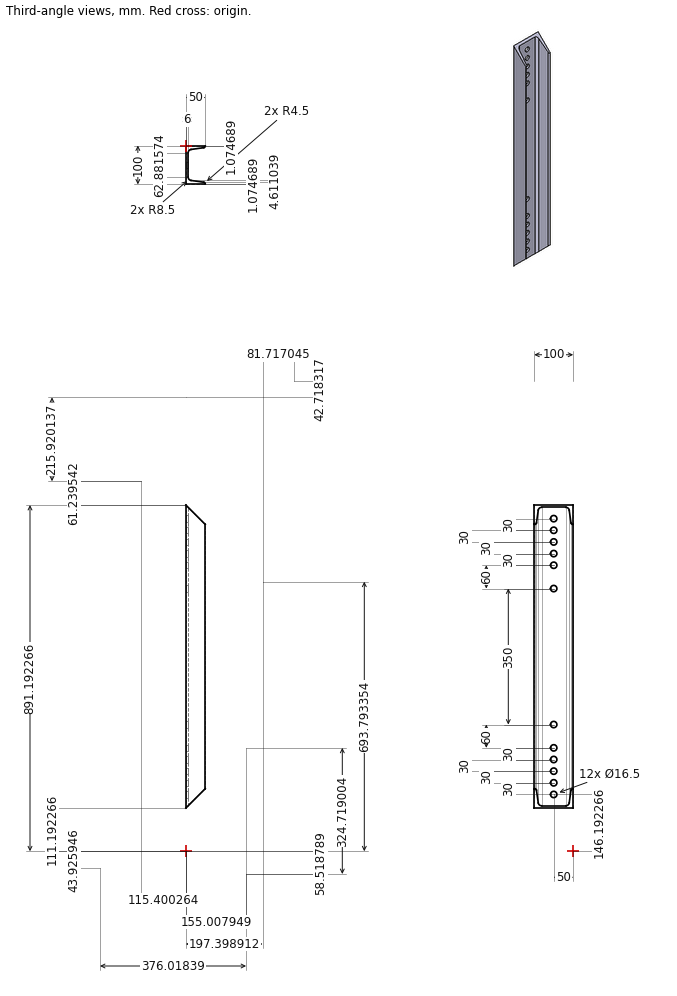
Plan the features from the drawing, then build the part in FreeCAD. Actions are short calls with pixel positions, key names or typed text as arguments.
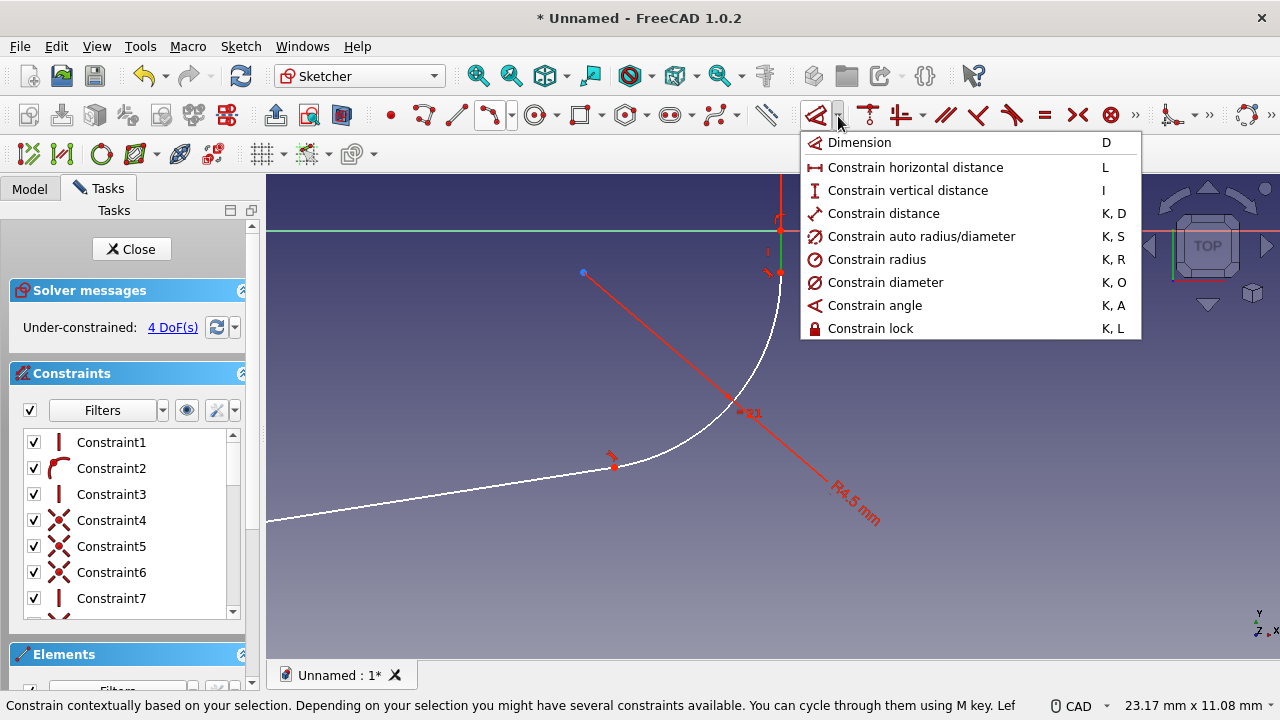
click(971, 190)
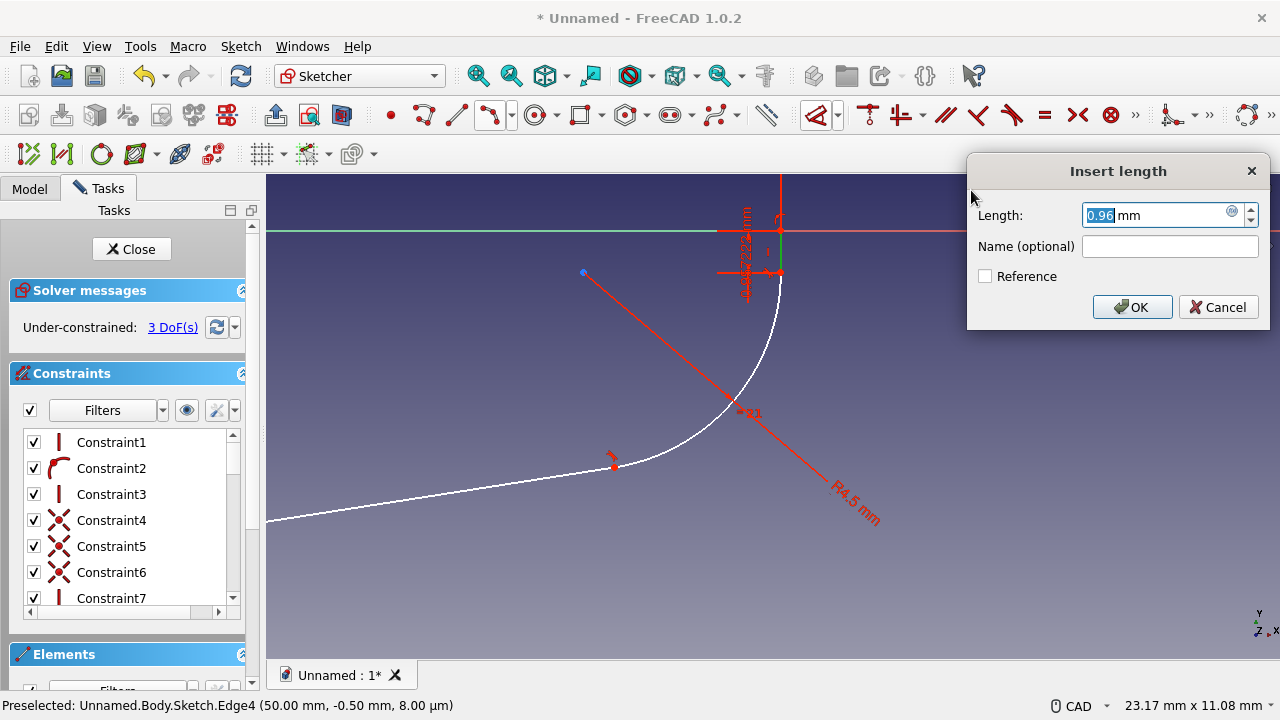
text(1.074689)
key(Return)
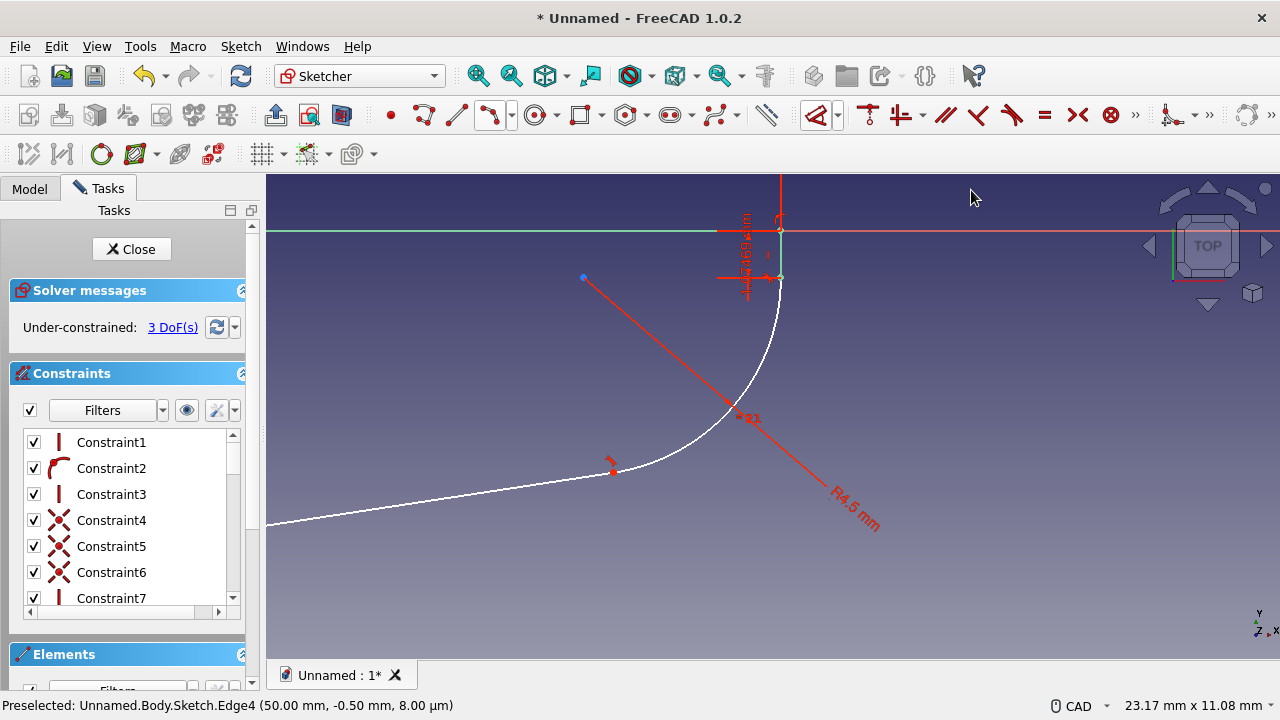
scroll(786, 256, down, 13)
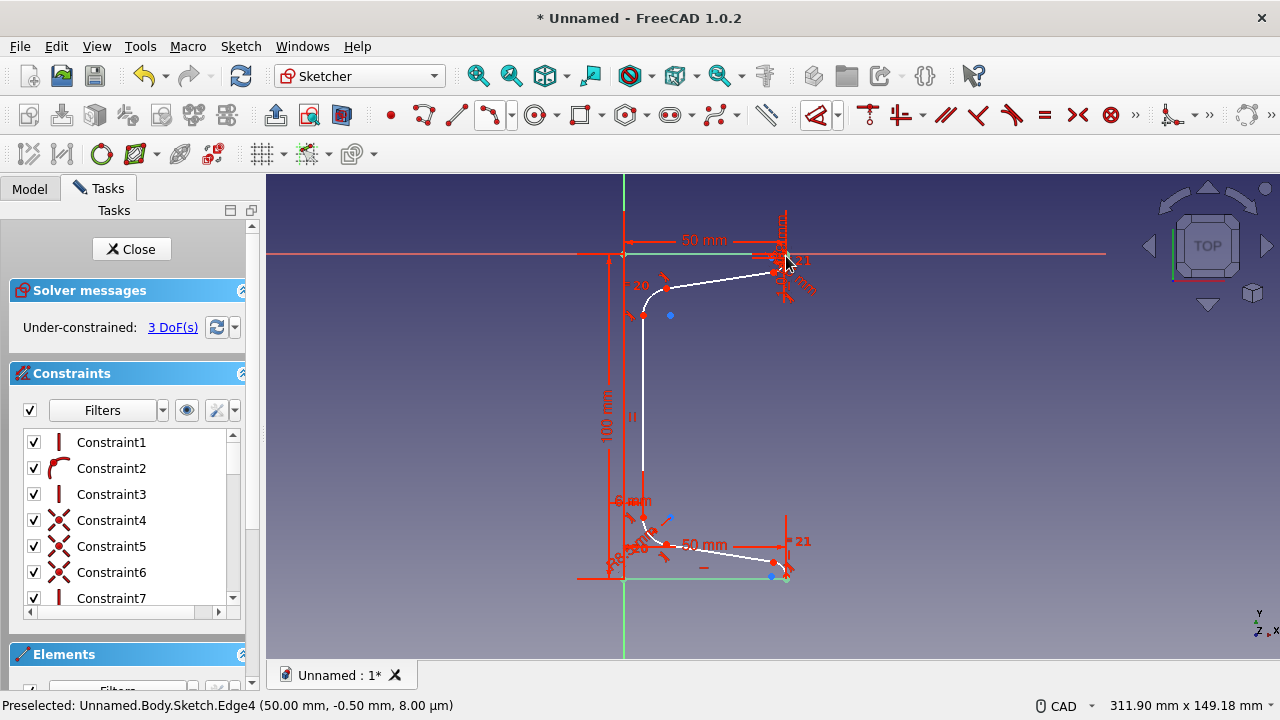
scroll(786, 579, up, 13)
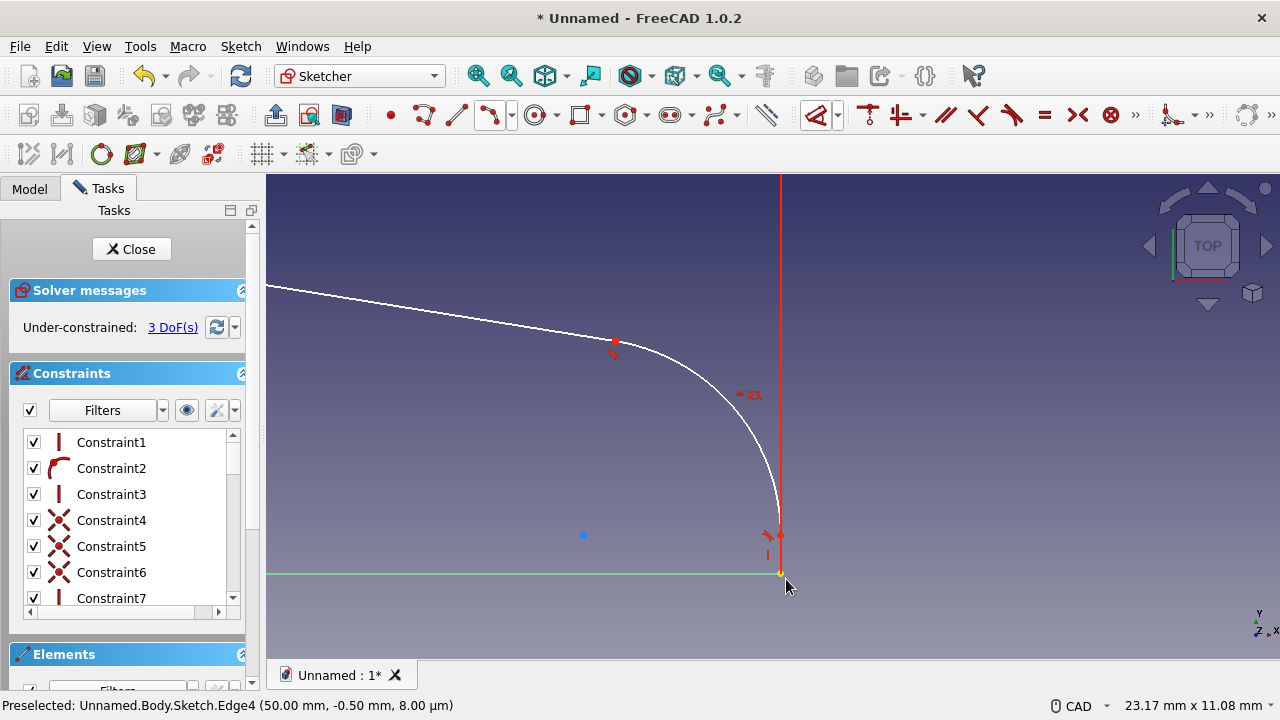
click(781, 562)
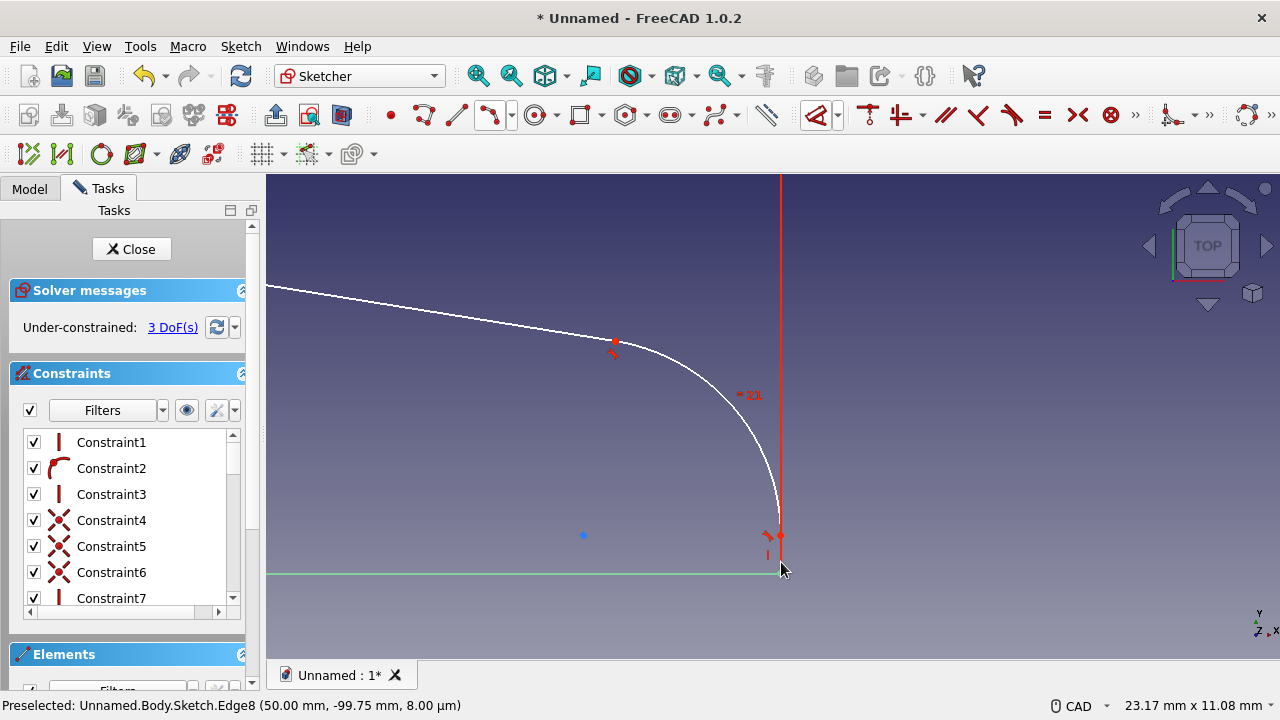
key(i)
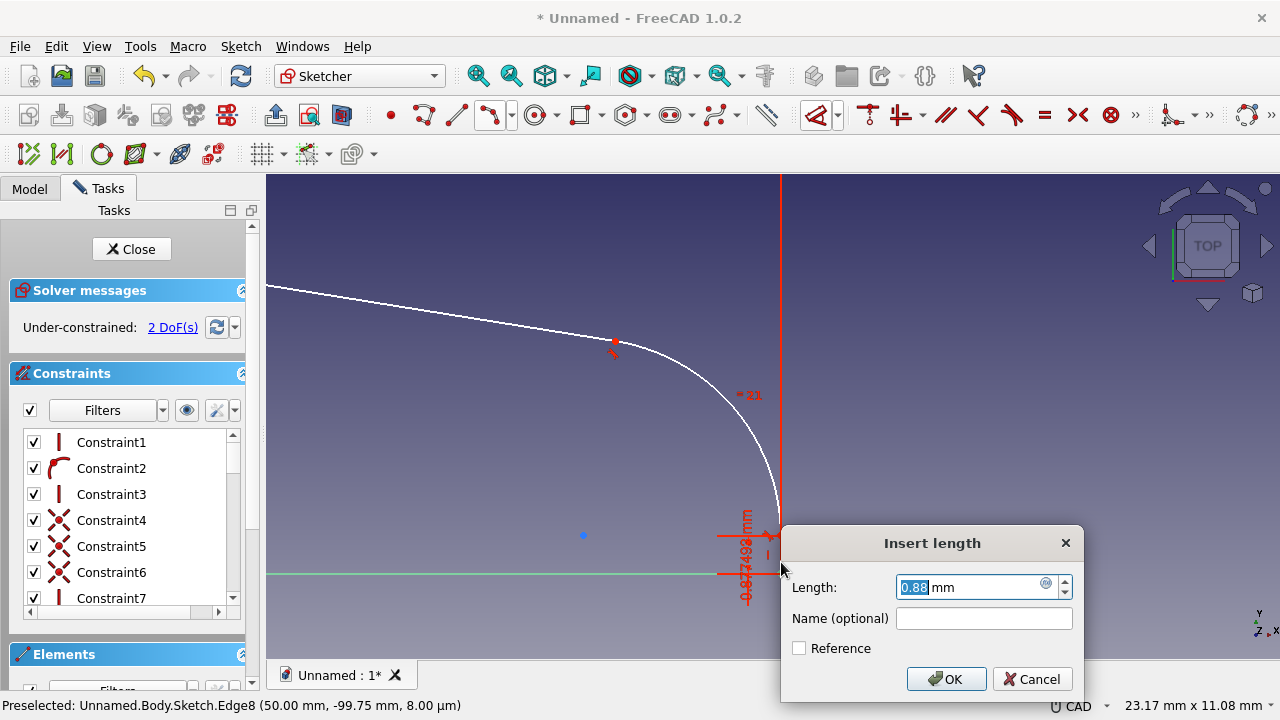
text(1.074689)
key(Return)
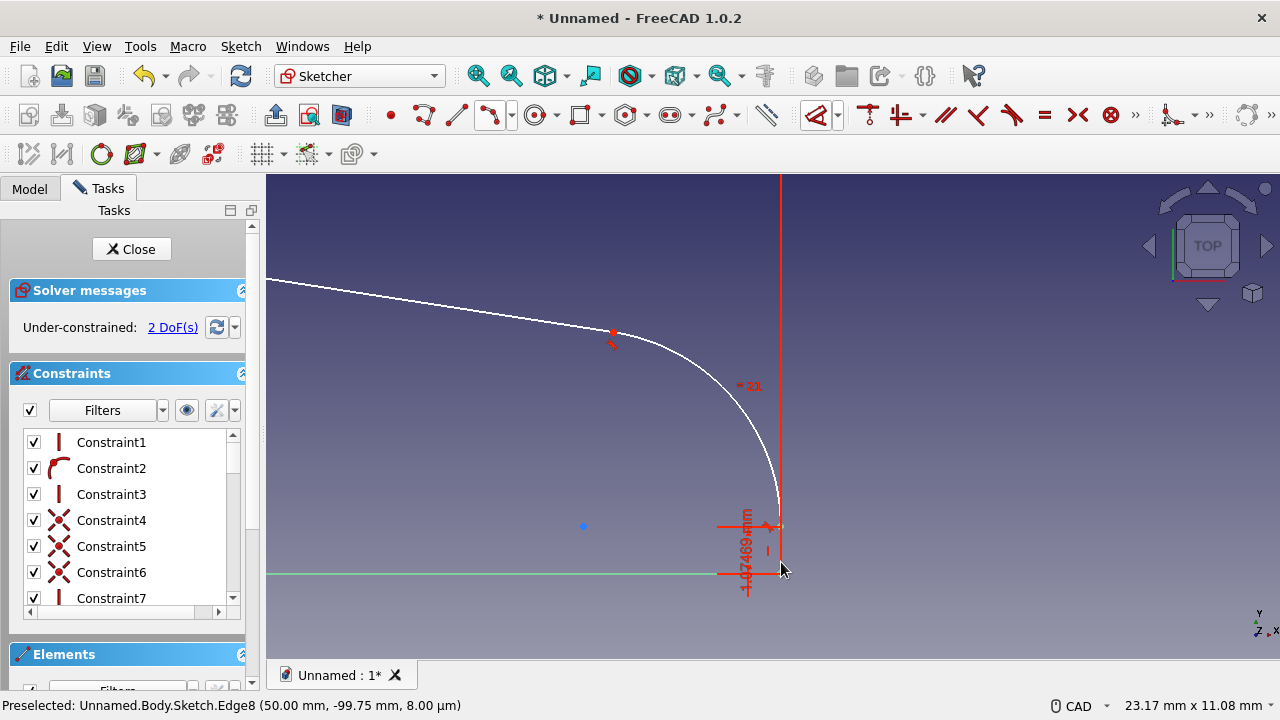
scroll(786, 579, down, 13)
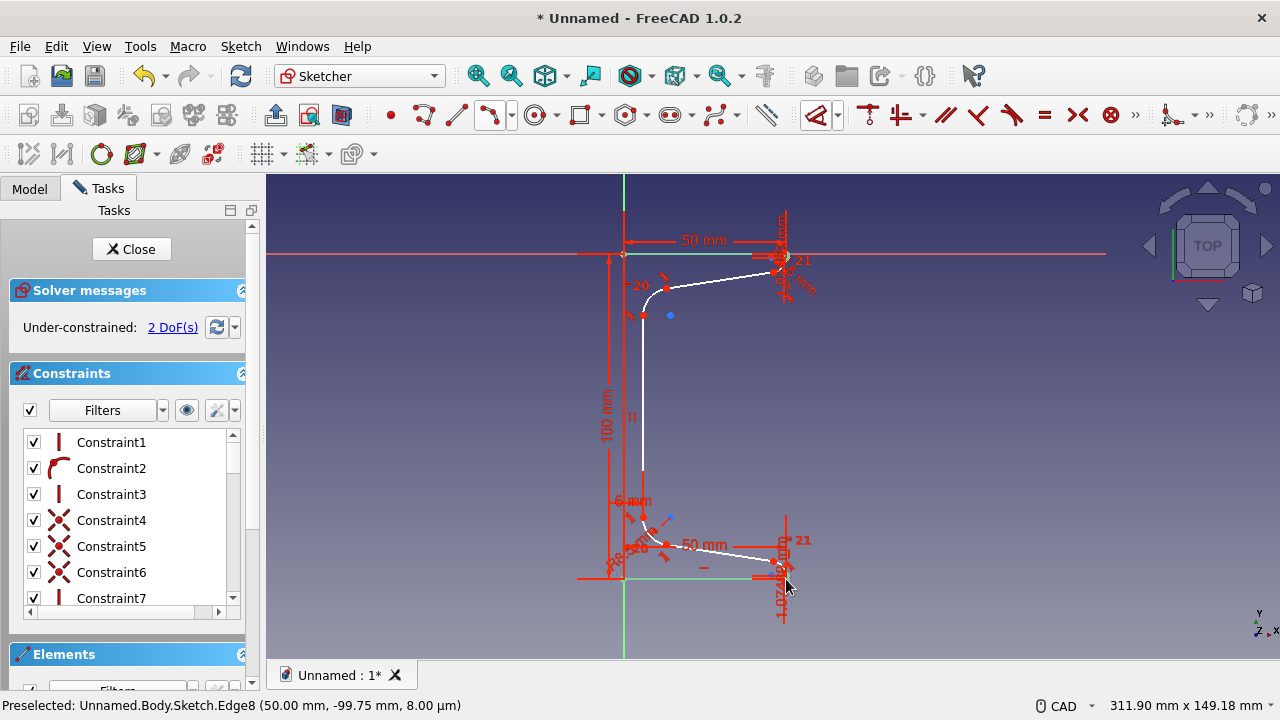
click(643, 457)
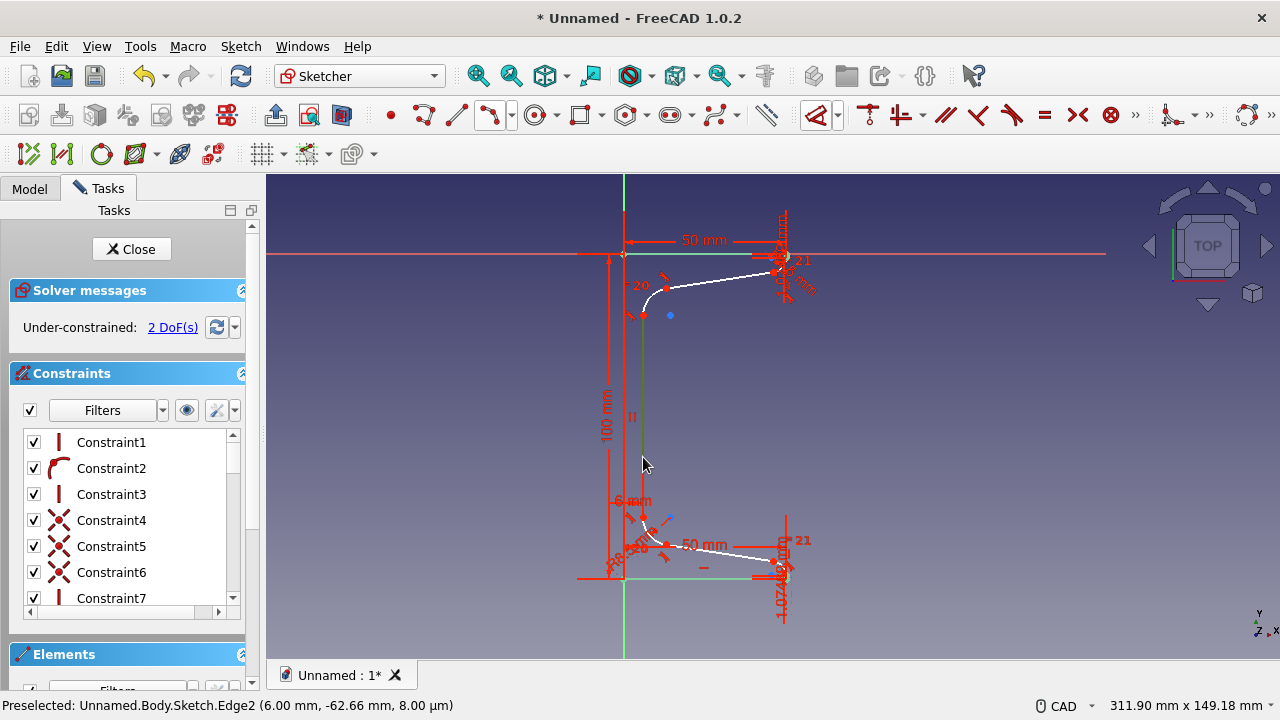
key(i)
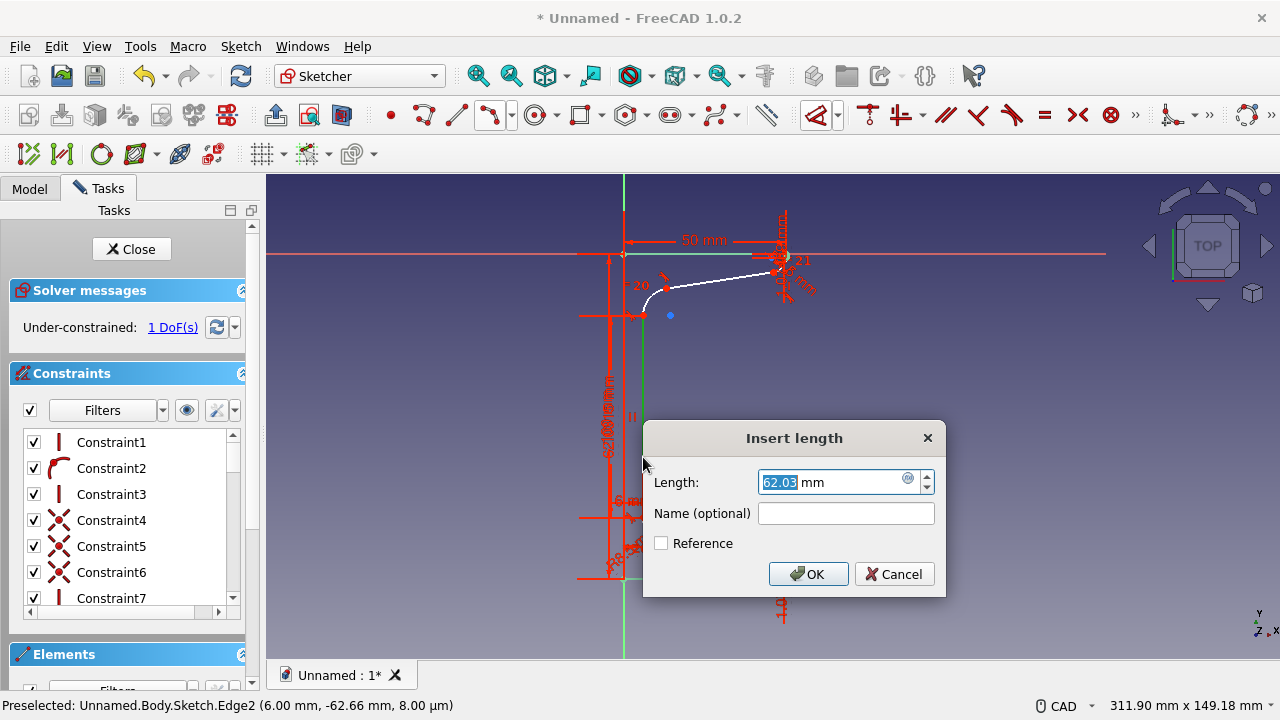
text(62.881574)
key(Return)